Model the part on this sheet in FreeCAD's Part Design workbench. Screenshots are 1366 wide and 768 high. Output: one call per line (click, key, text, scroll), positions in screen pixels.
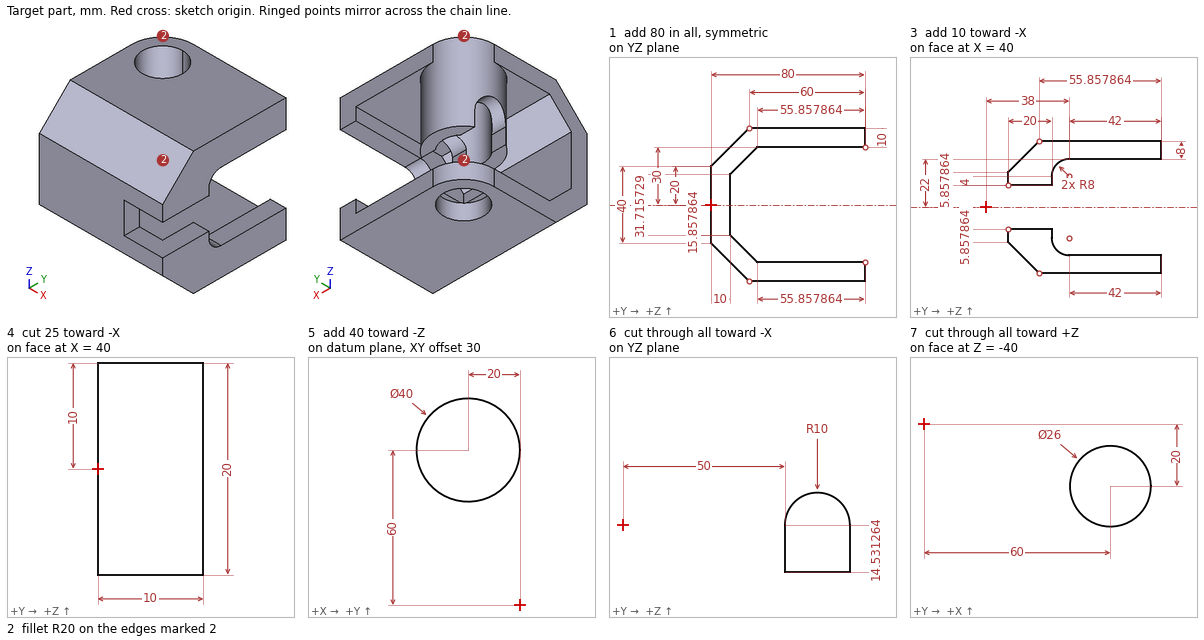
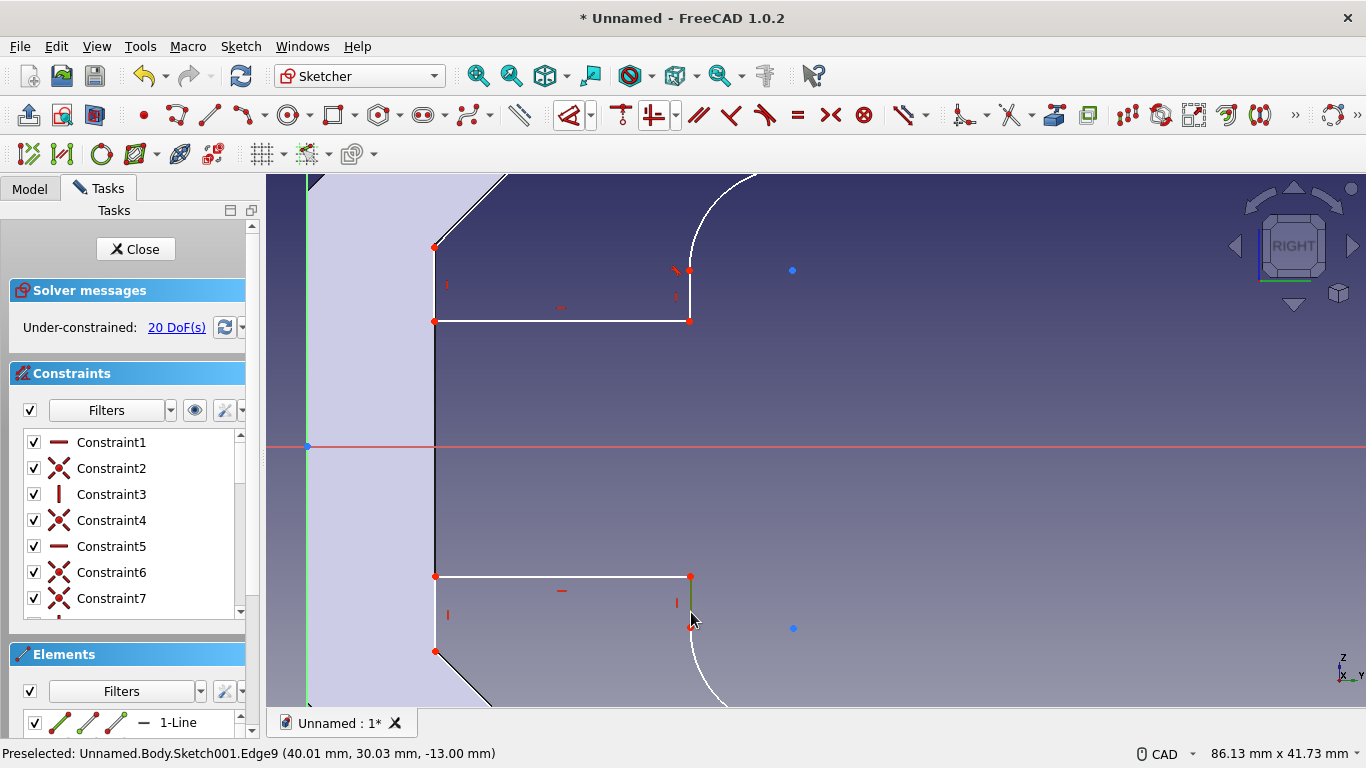
click(701, 674)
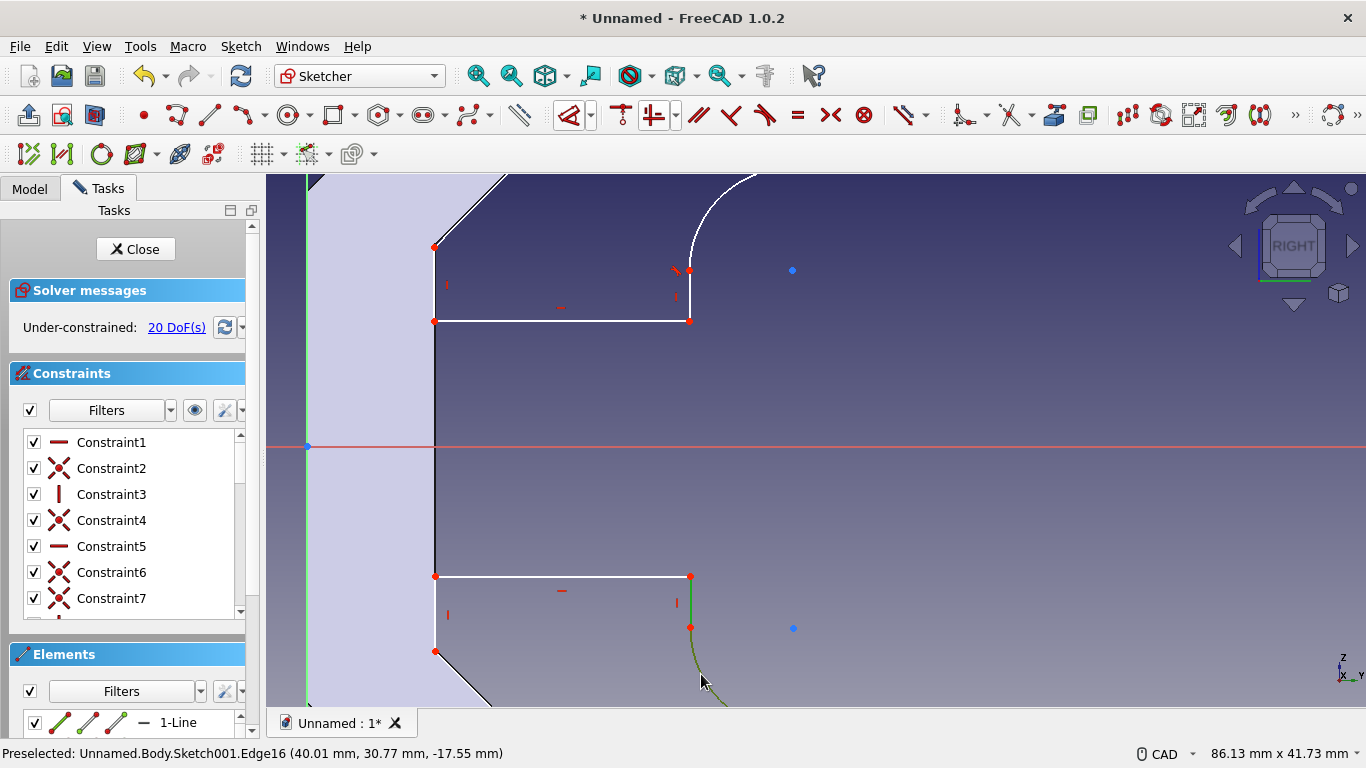
click(765, 116)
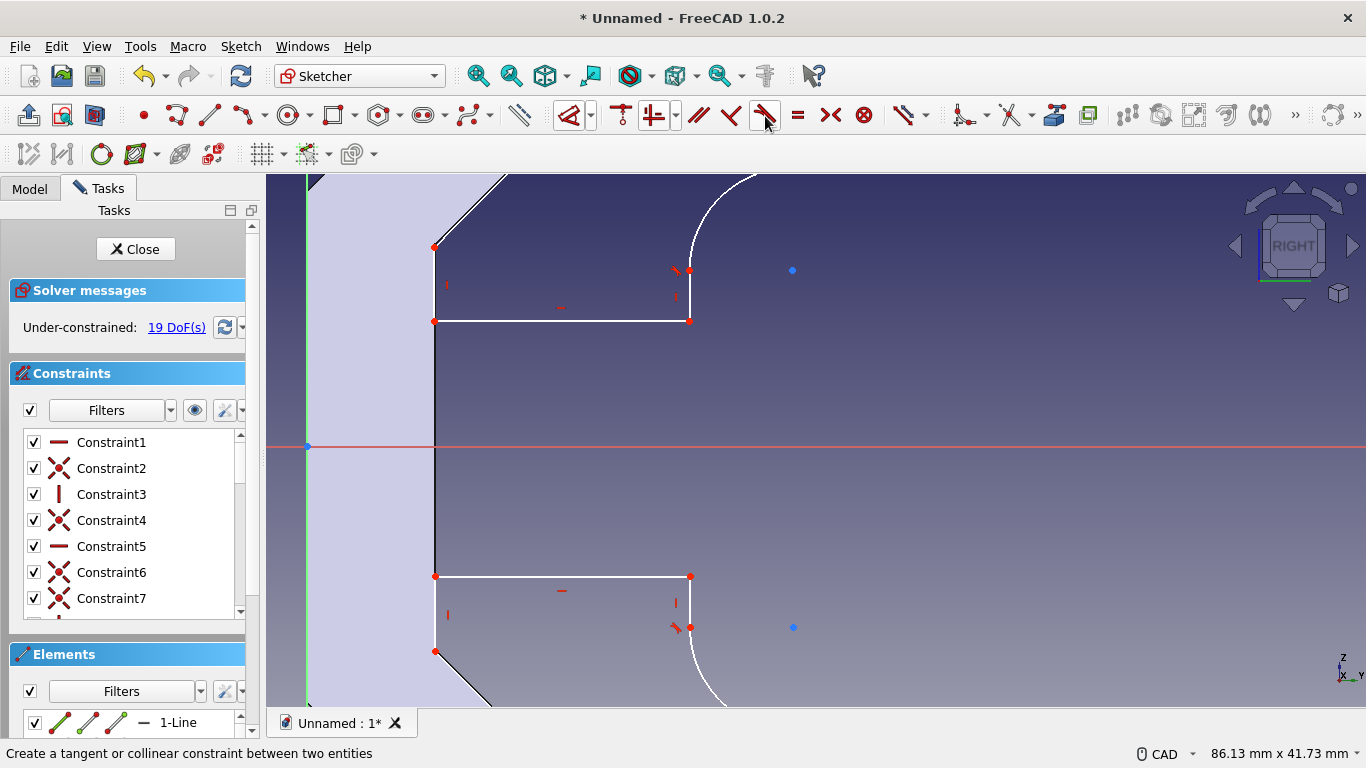
scroll(690, 435, down, 4)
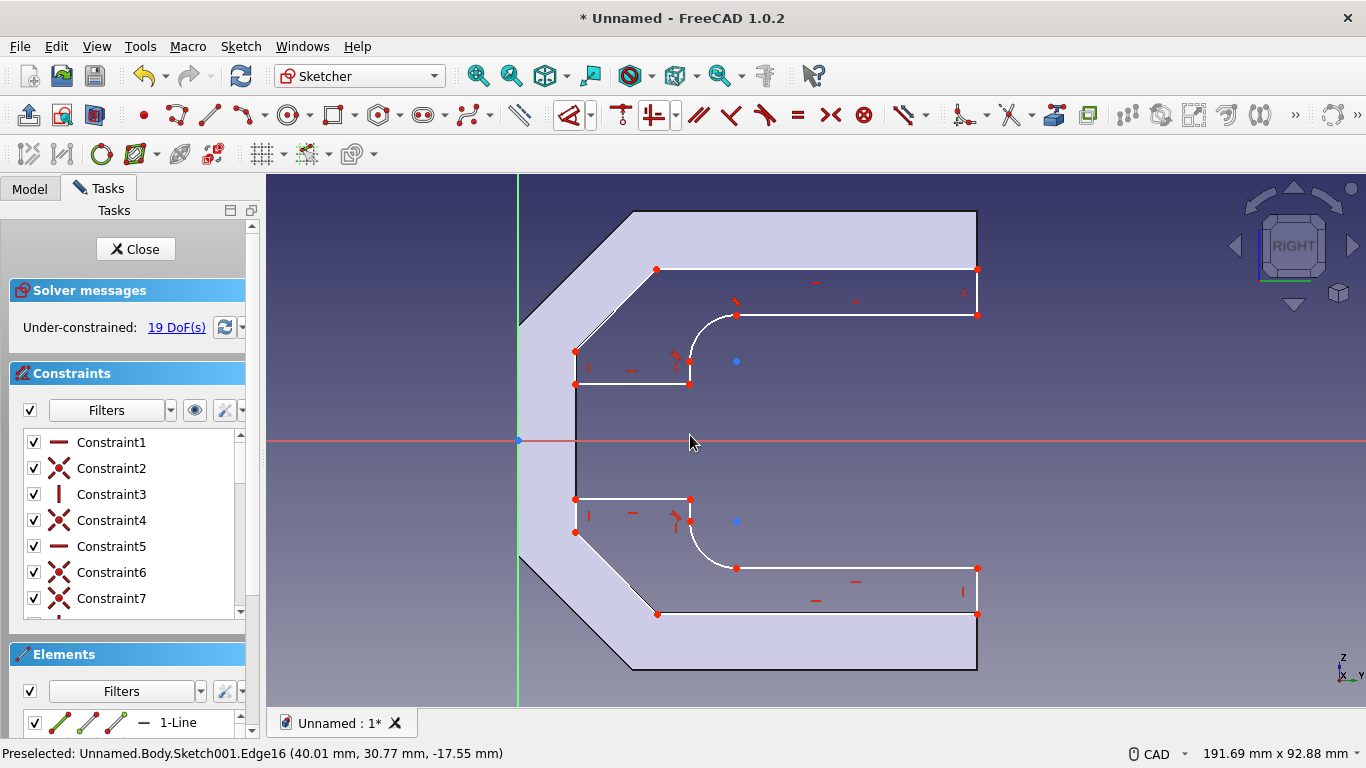
click(905, 568)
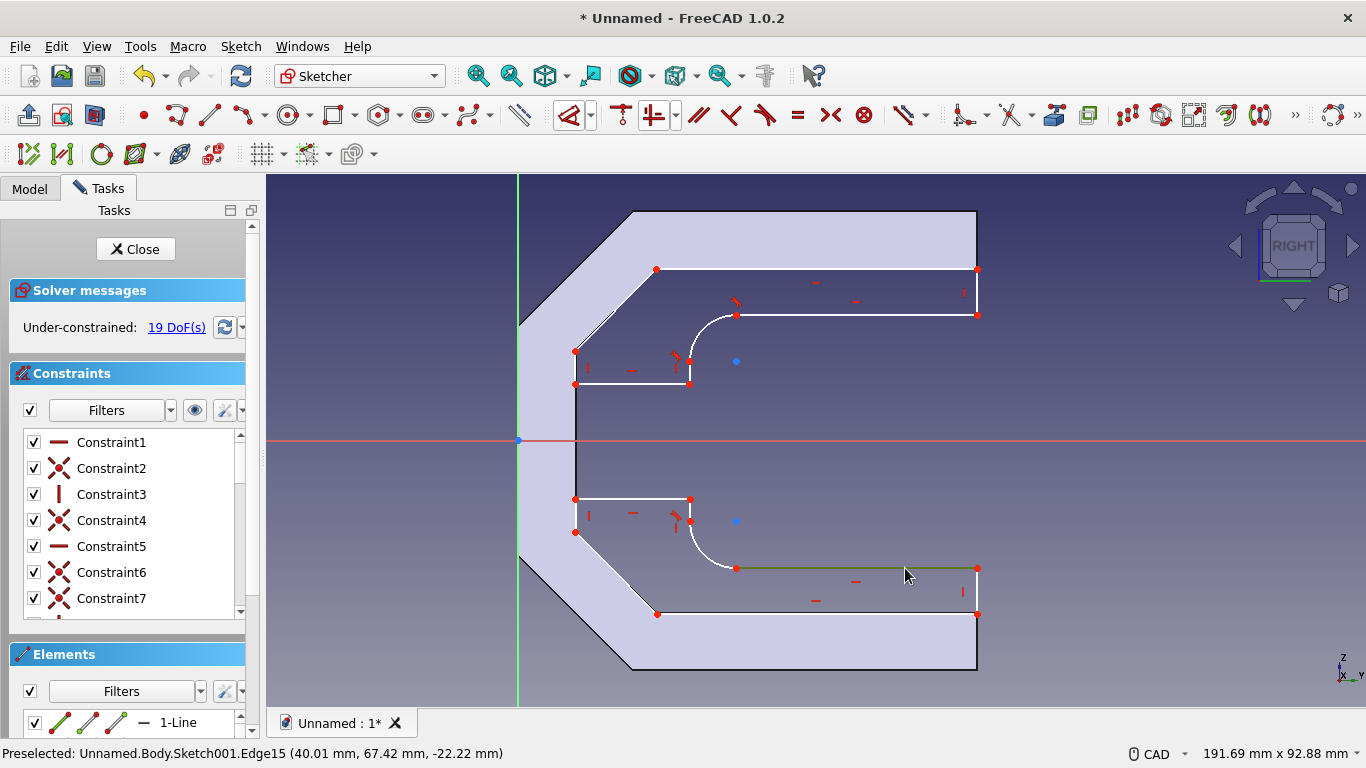
click(695, 543)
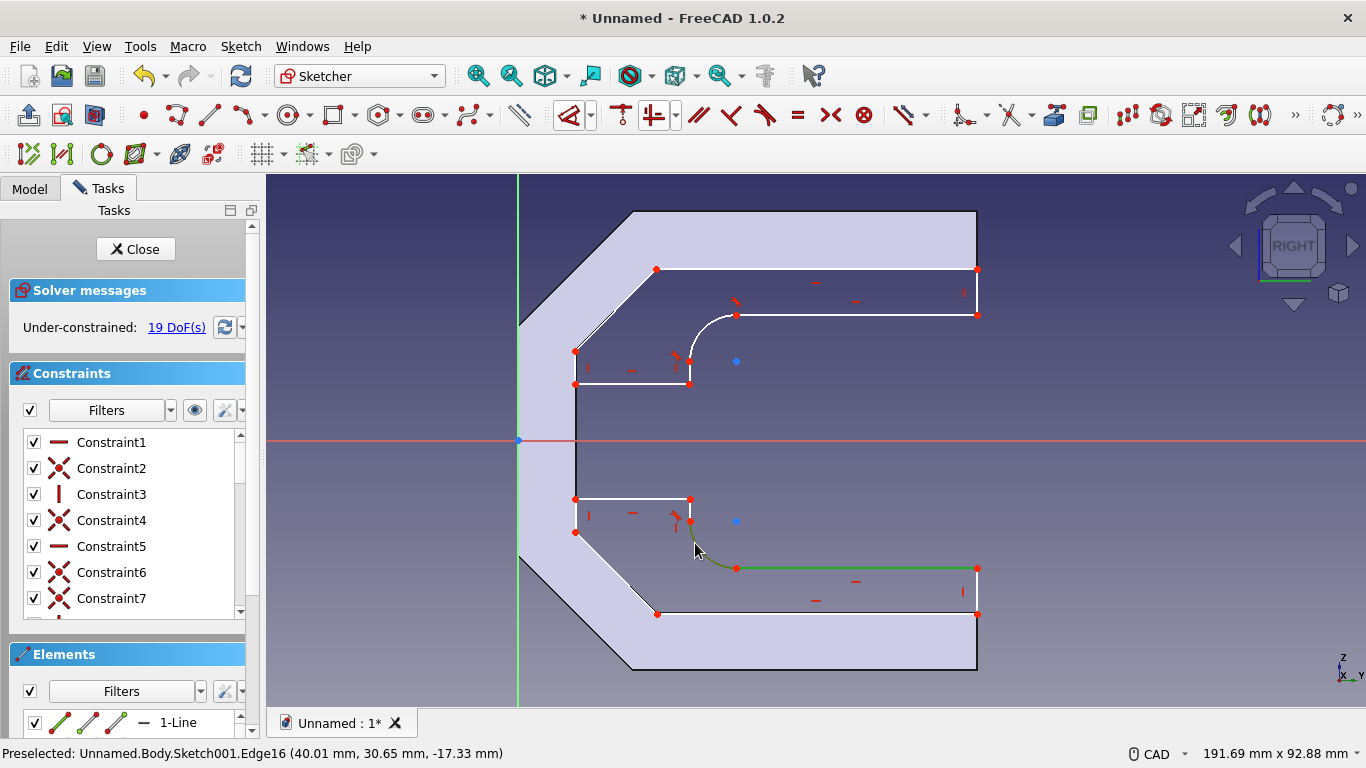
click(765, 116)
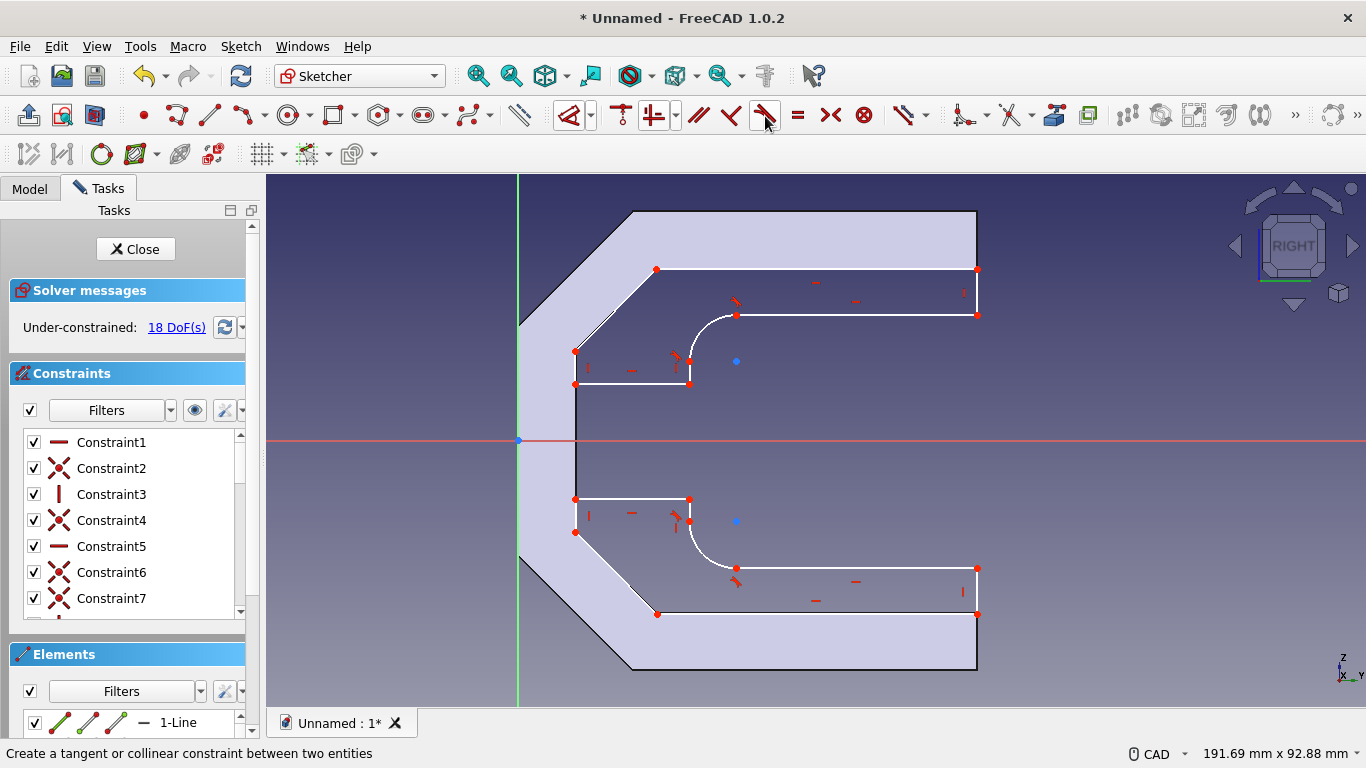
click(715, 320)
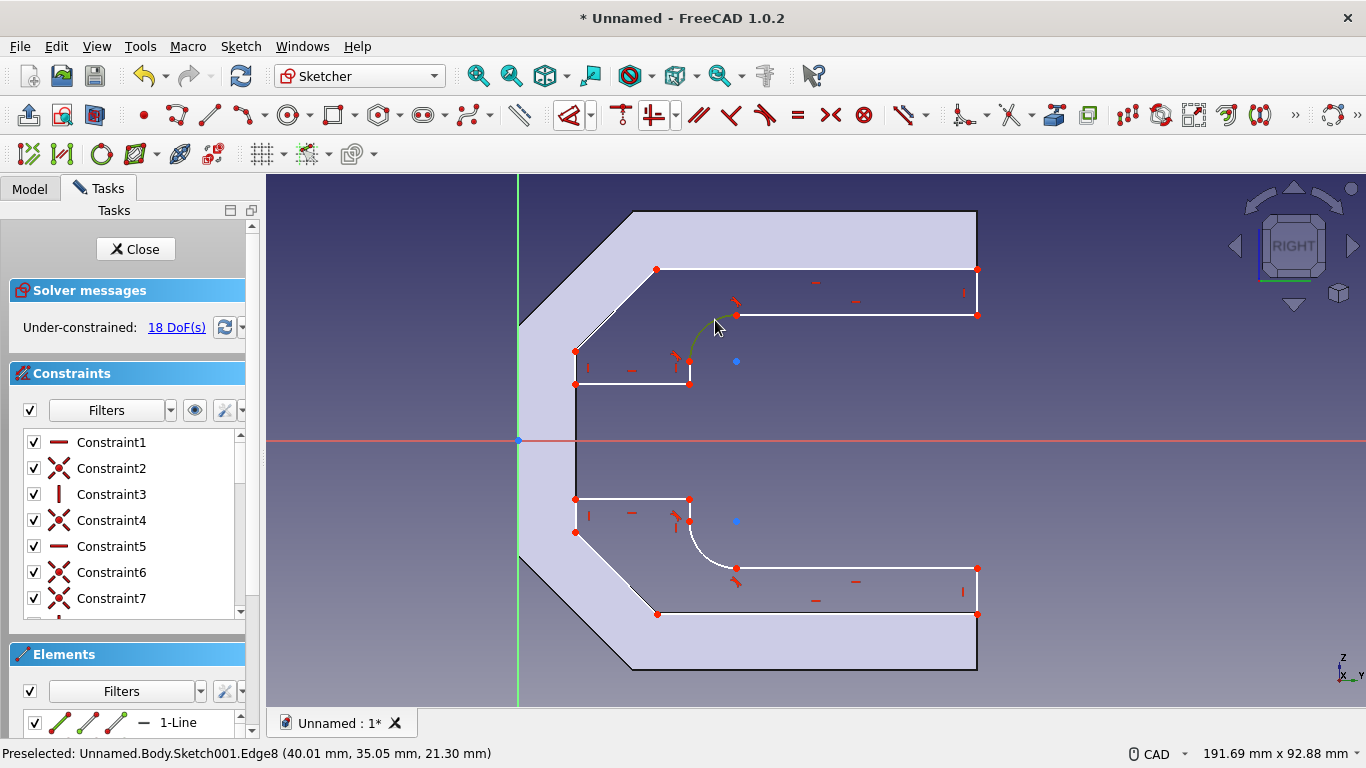
click(695, 543)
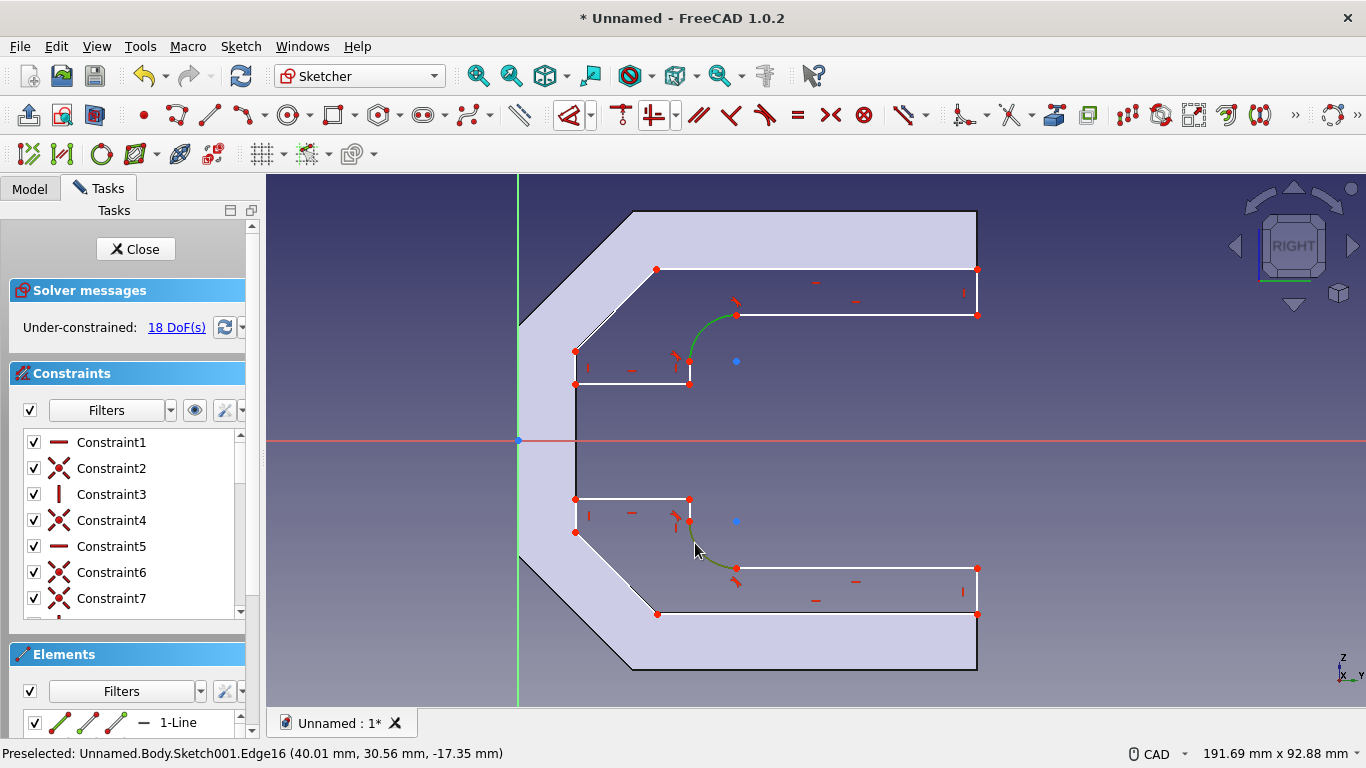
click(798, 116)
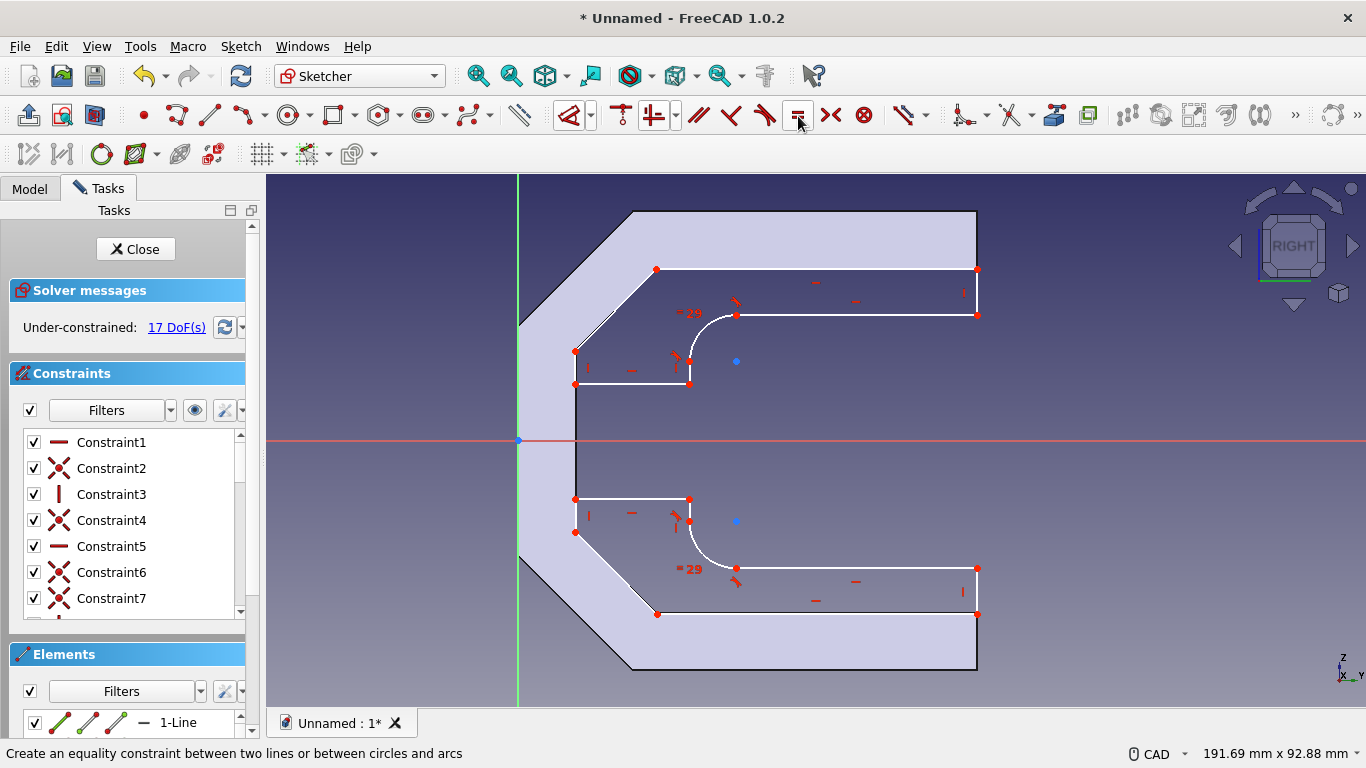
click(736, 361)